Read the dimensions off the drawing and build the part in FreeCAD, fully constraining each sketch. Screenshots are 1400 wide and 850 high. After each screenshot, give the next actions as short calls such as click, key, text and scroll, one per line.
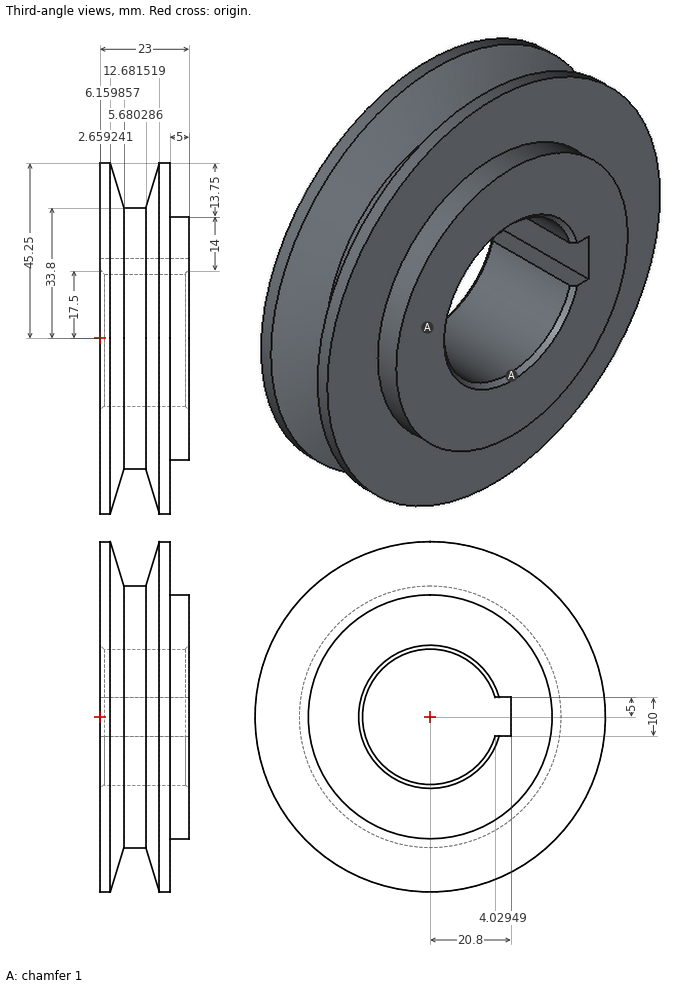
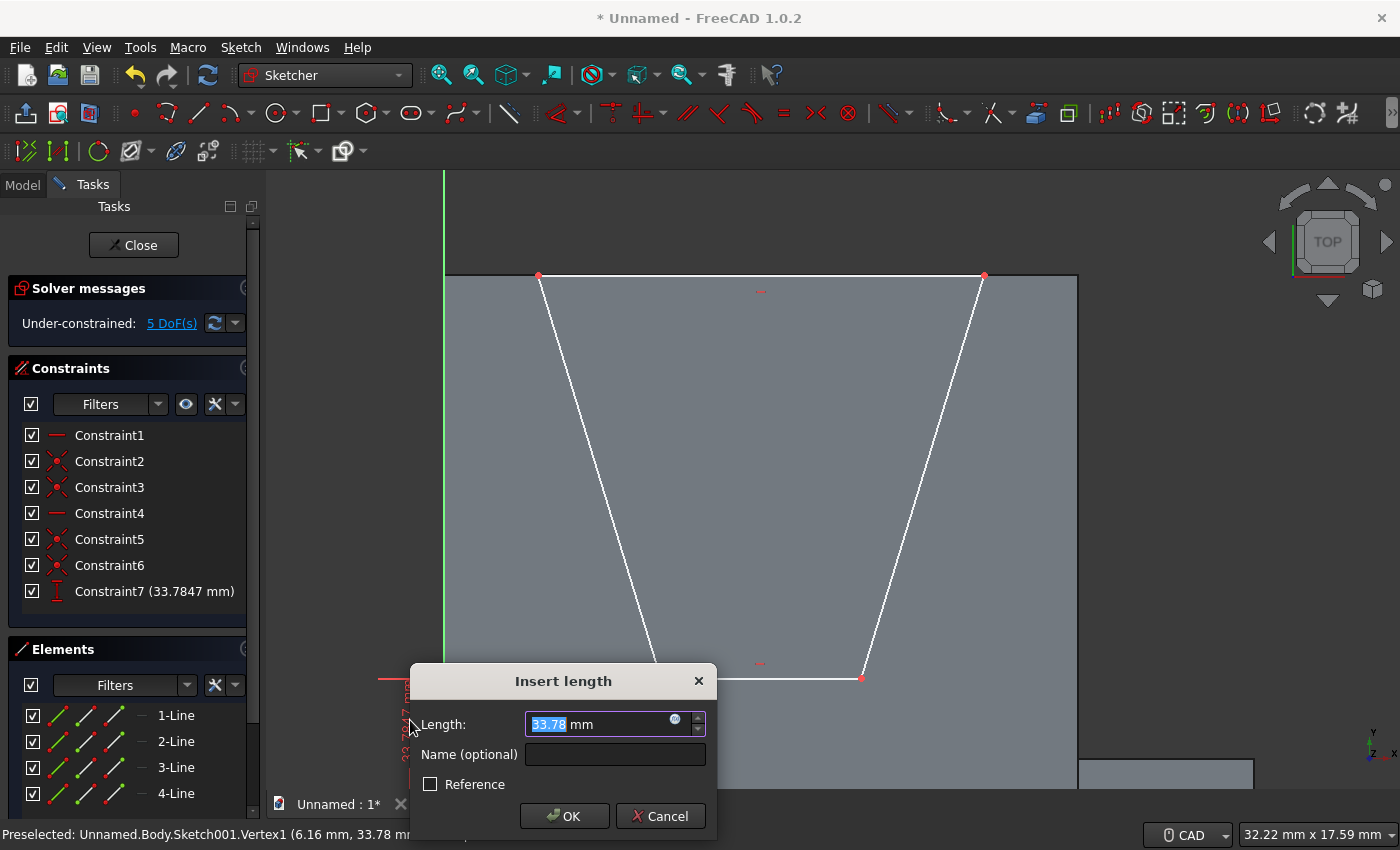
text(33.8)
key(Return)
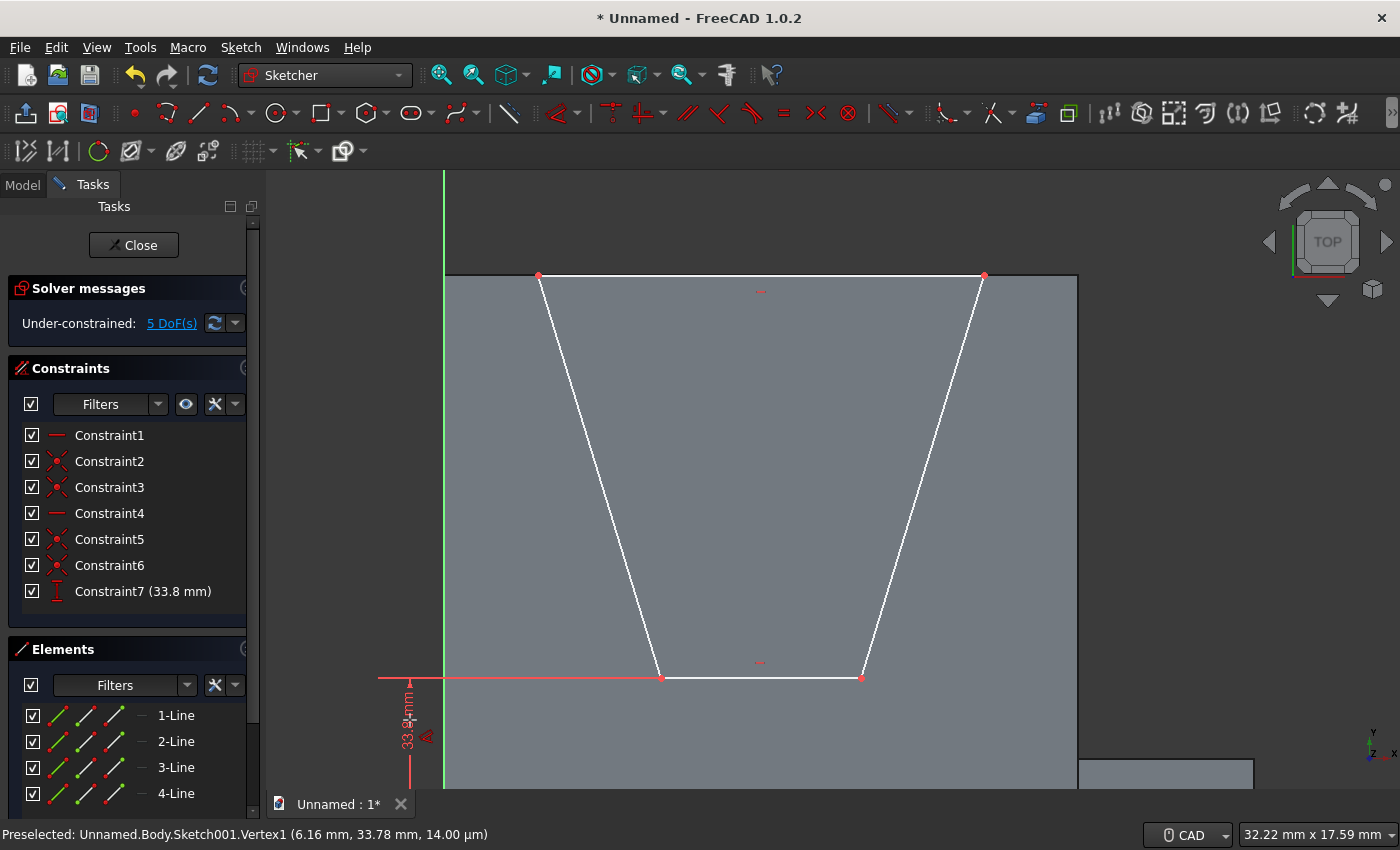
click(984, 276)
click(410, 518)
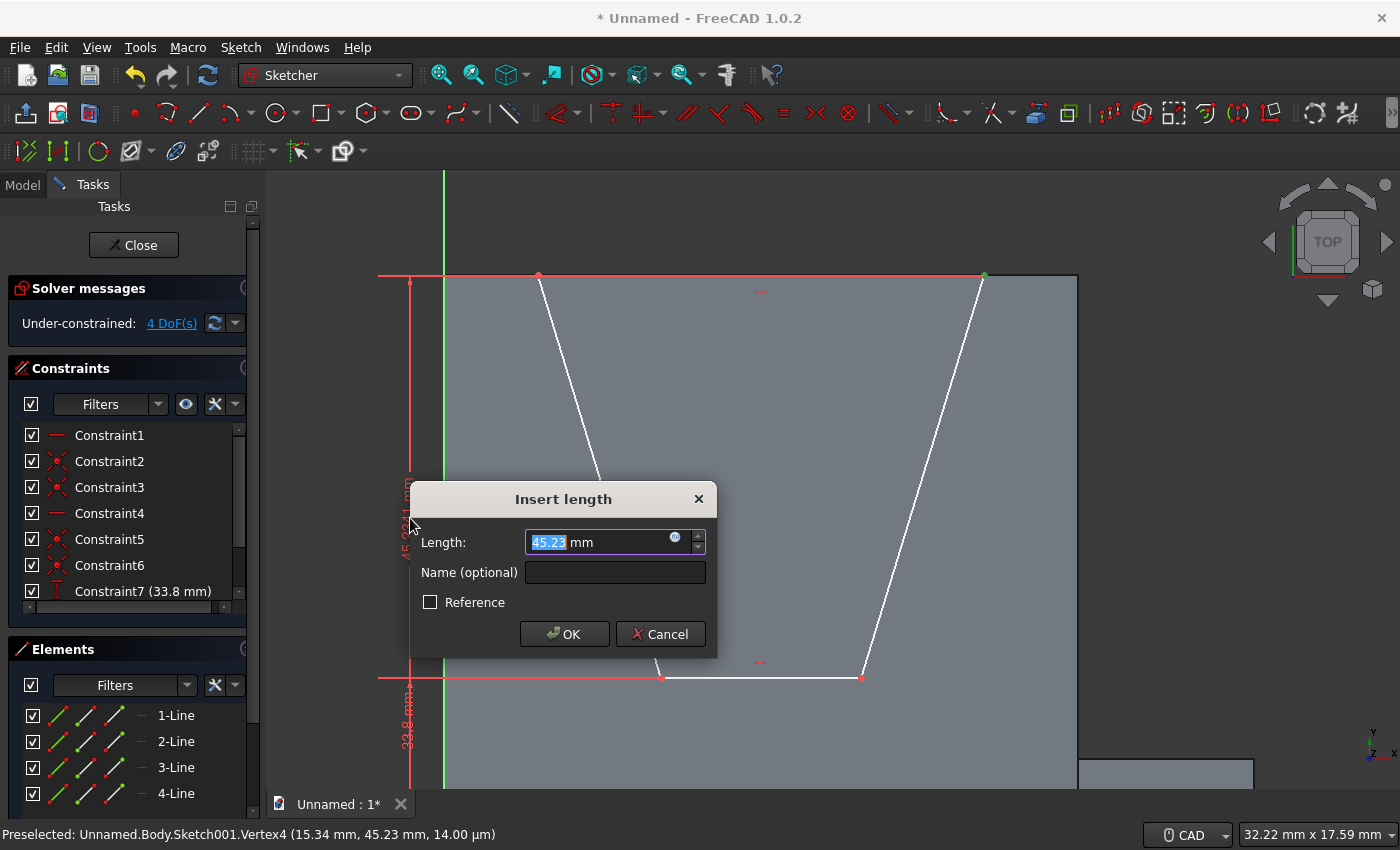
text(45.25)
key(Return)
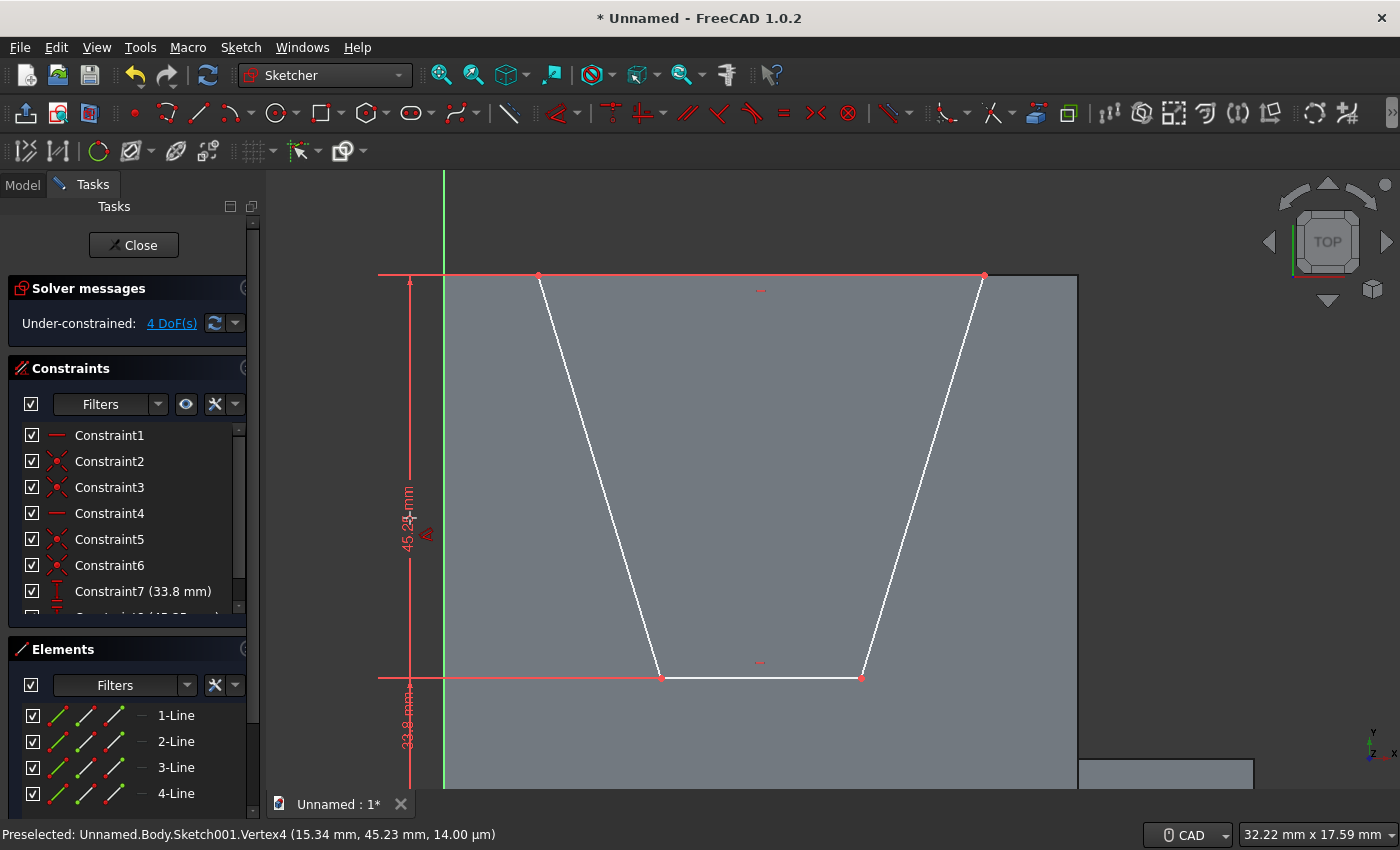
click(721, 678)
click(761, 712)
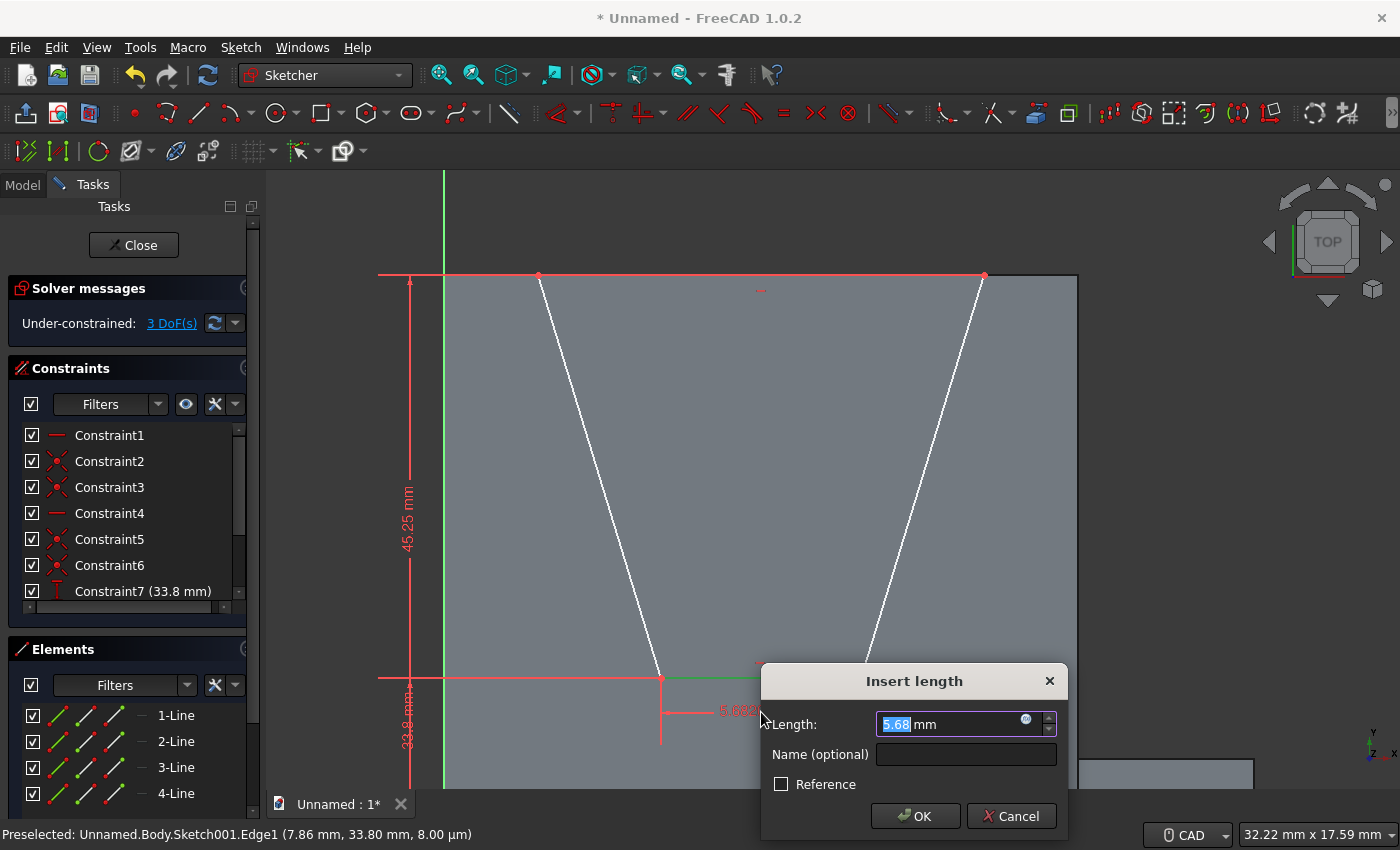
text(5.680286)
key(Return)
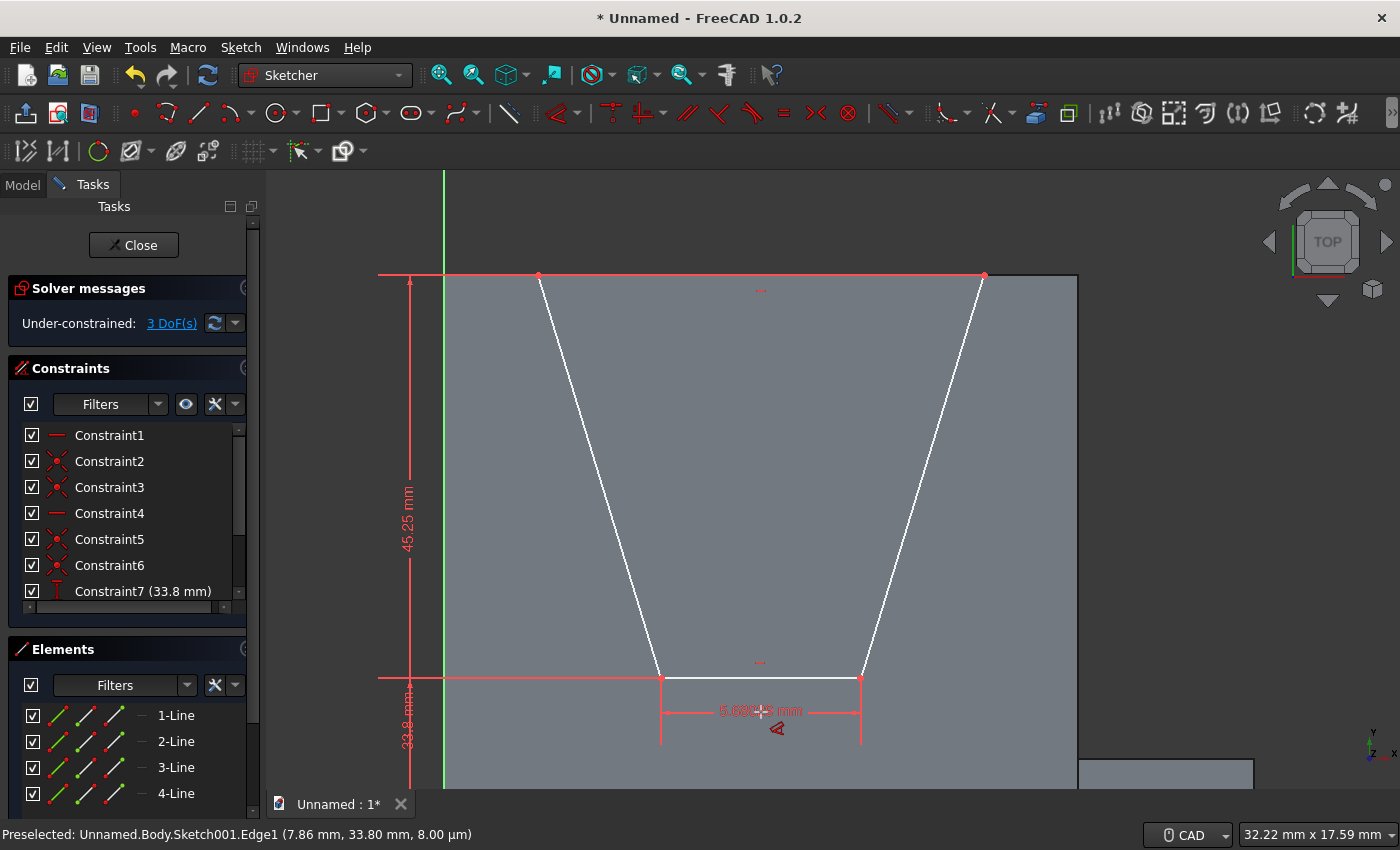
click(850, 275)
click(761, 241)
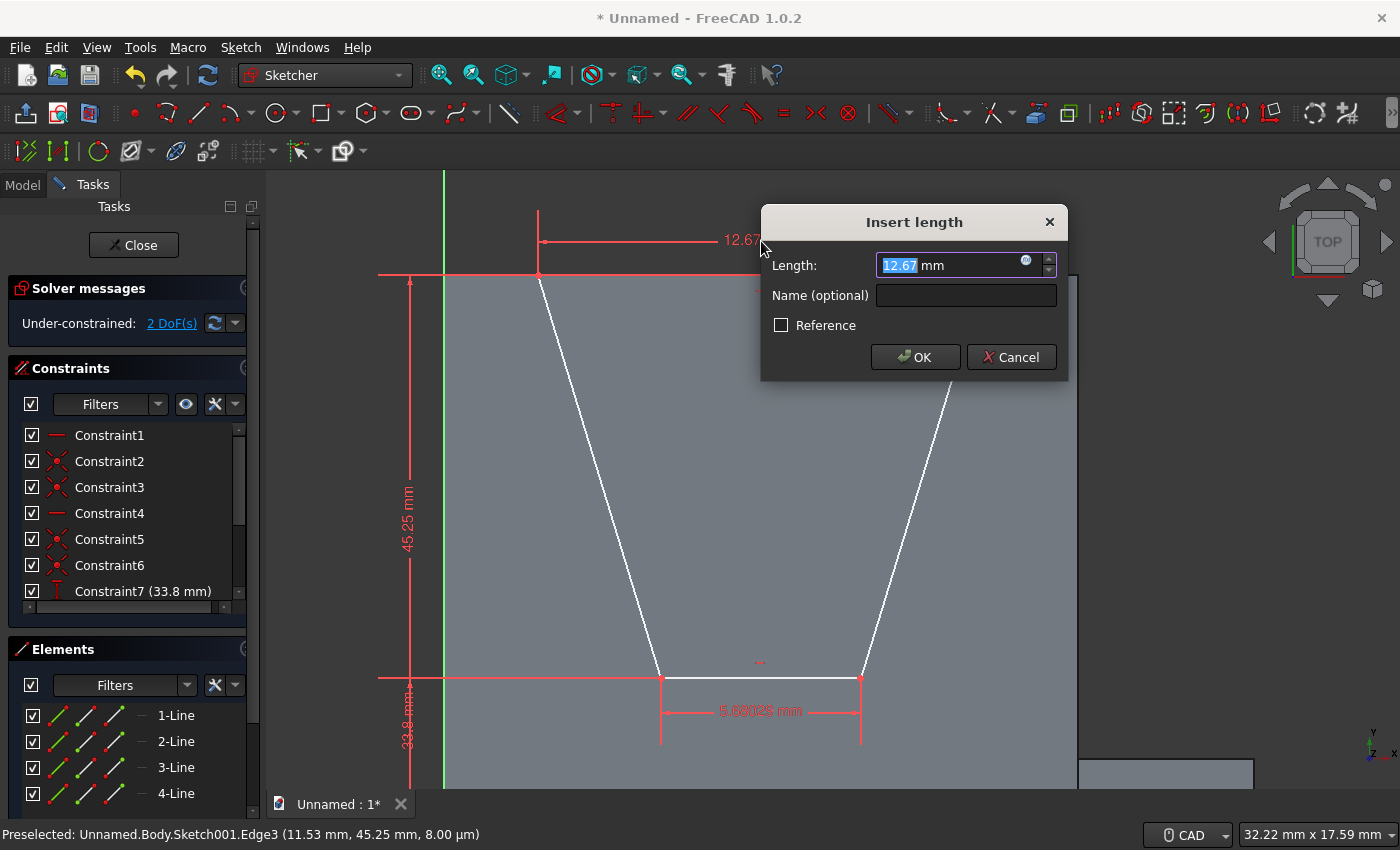
text(12.681519)
key(Return)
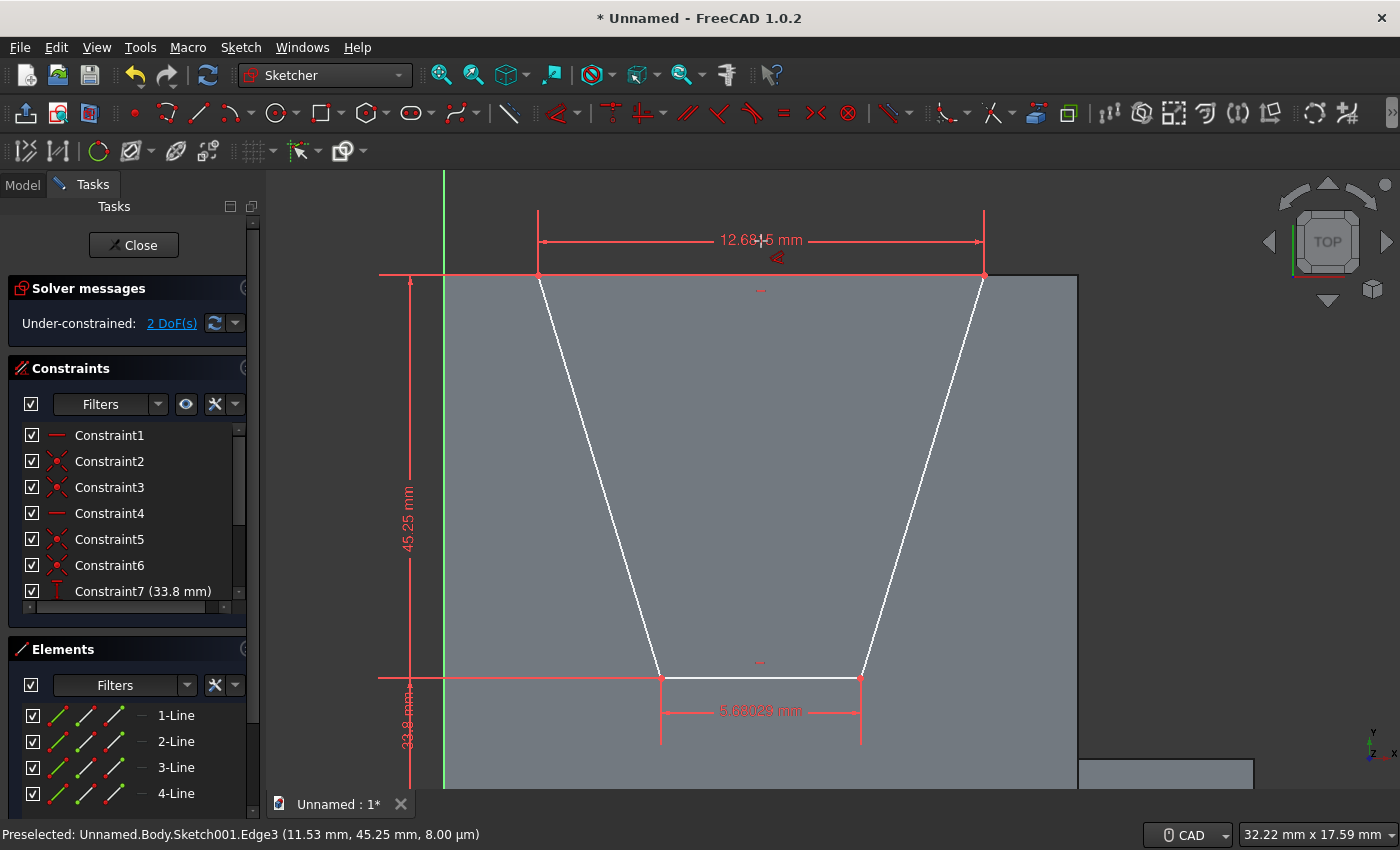
click(661, 678)
click(553, 644)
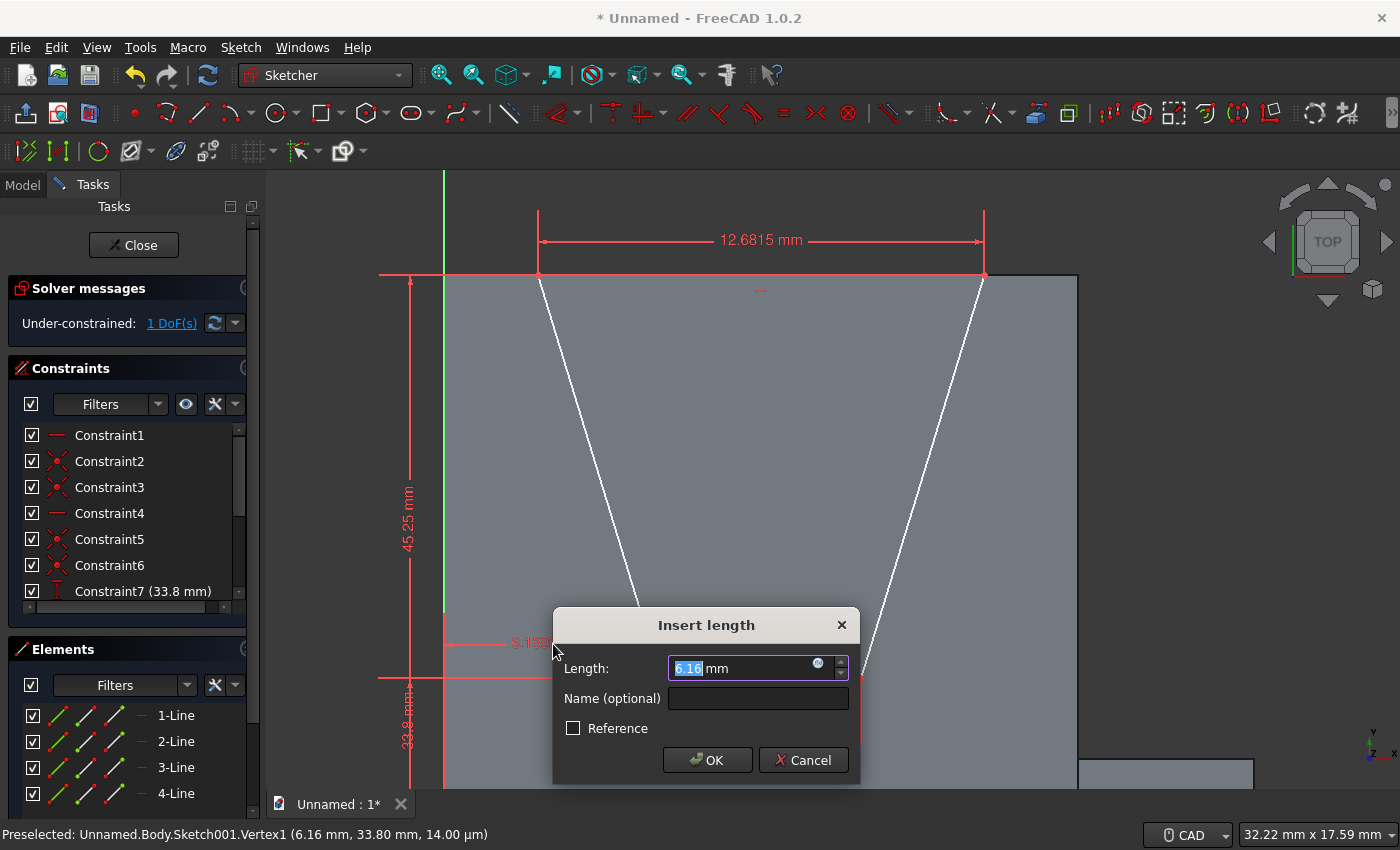
text(6.159857)
key(Return)